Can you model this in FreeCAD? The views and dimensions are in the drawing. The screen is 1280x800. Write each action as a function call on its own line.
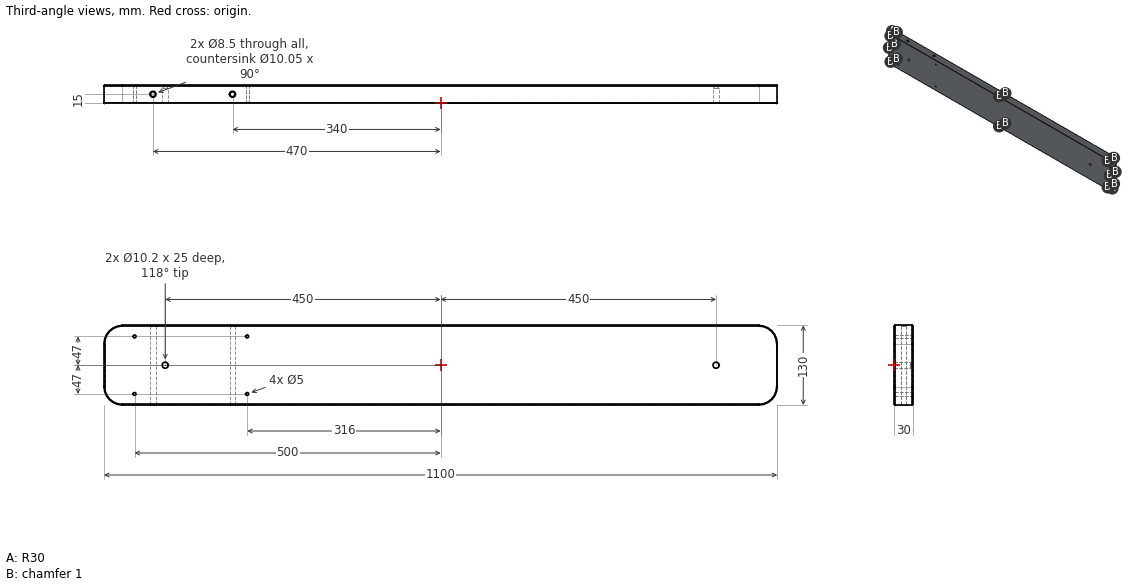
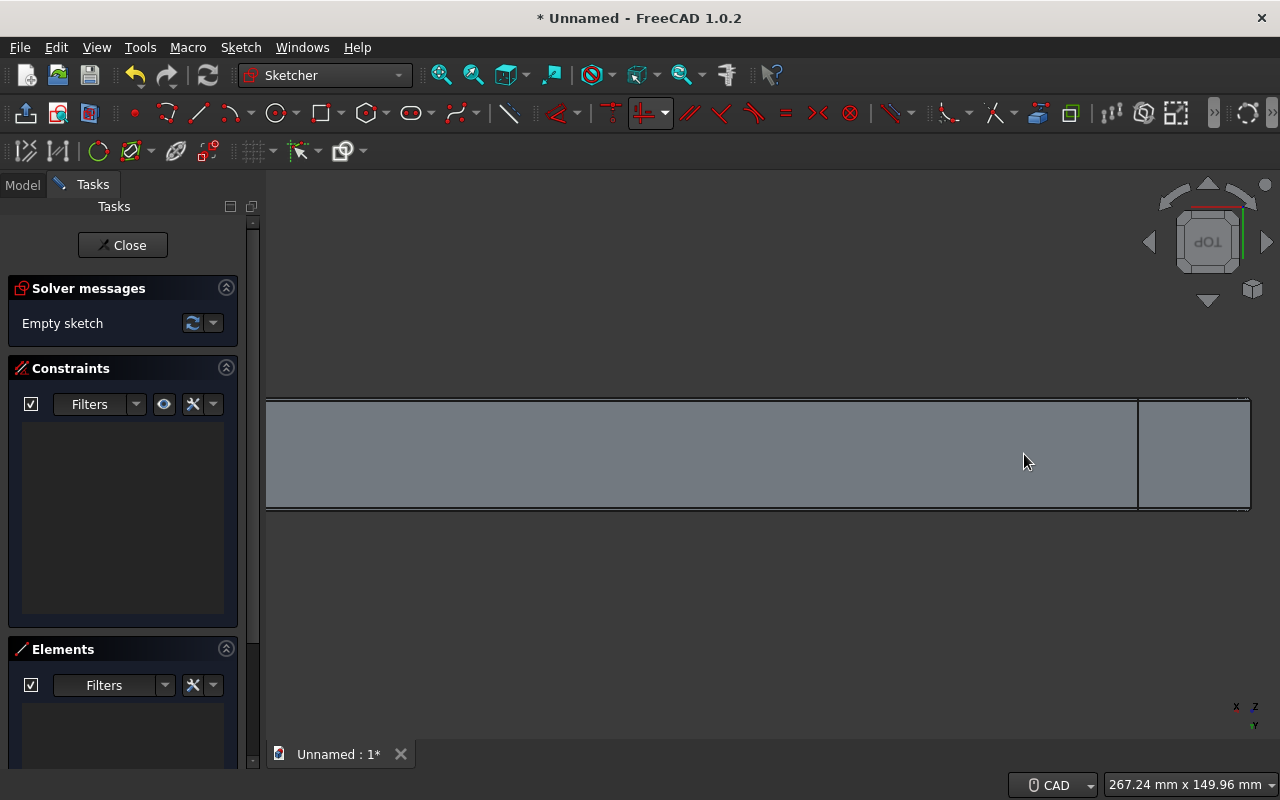
click(276, 114)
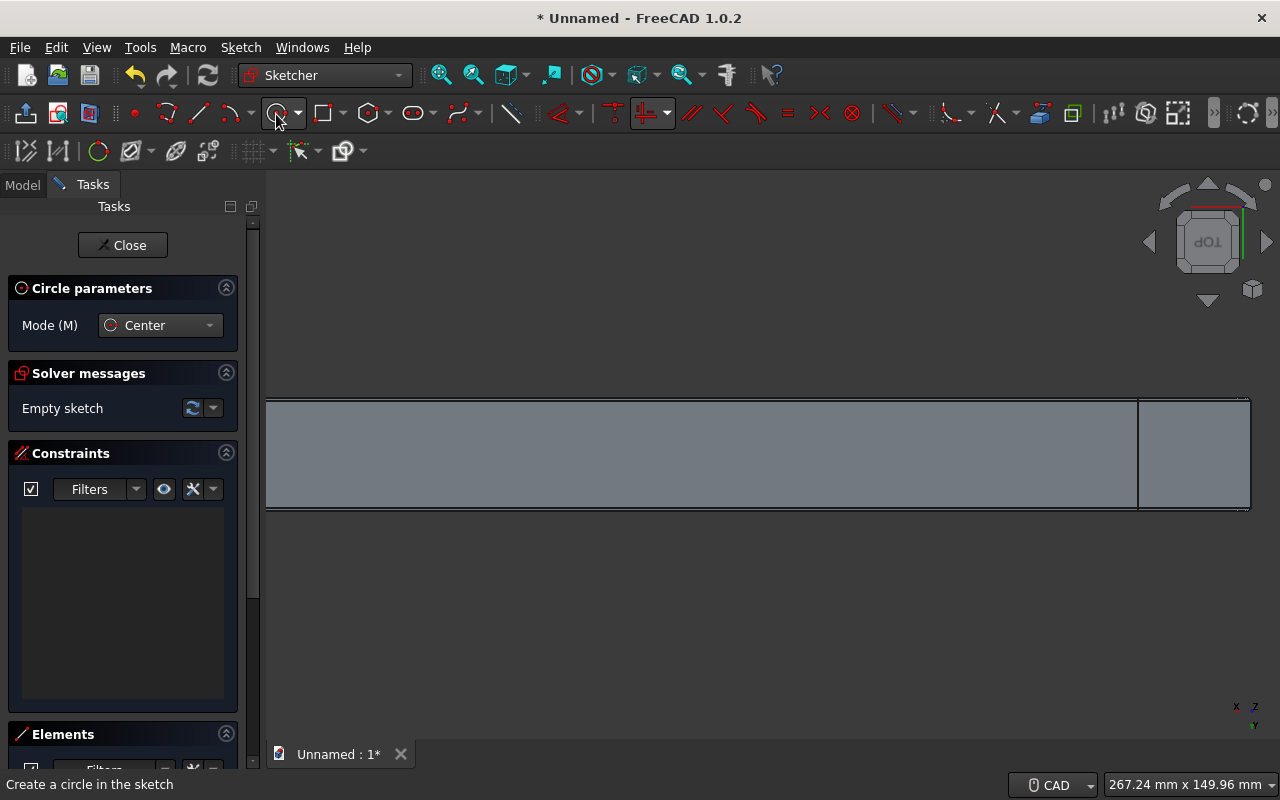
scroll(948, 455, up, 2)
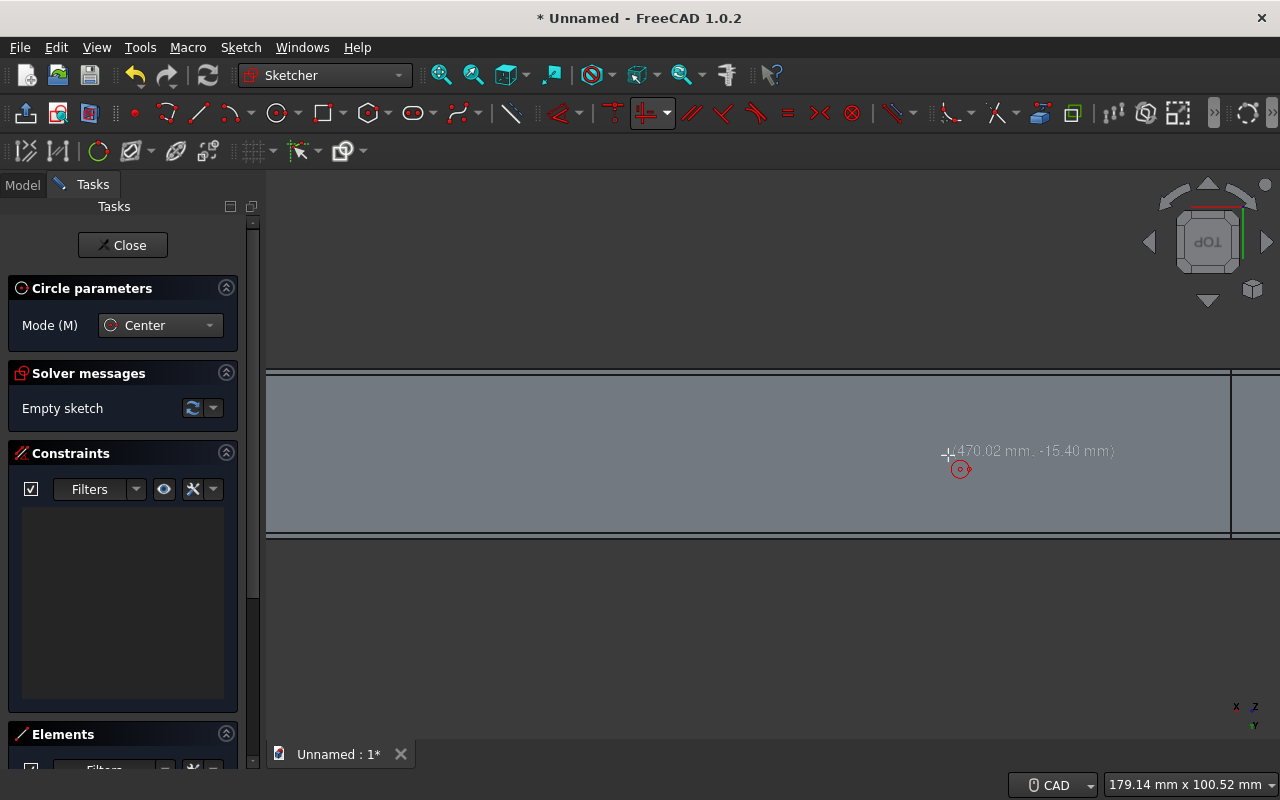
click(948, 454)
click(965, 437)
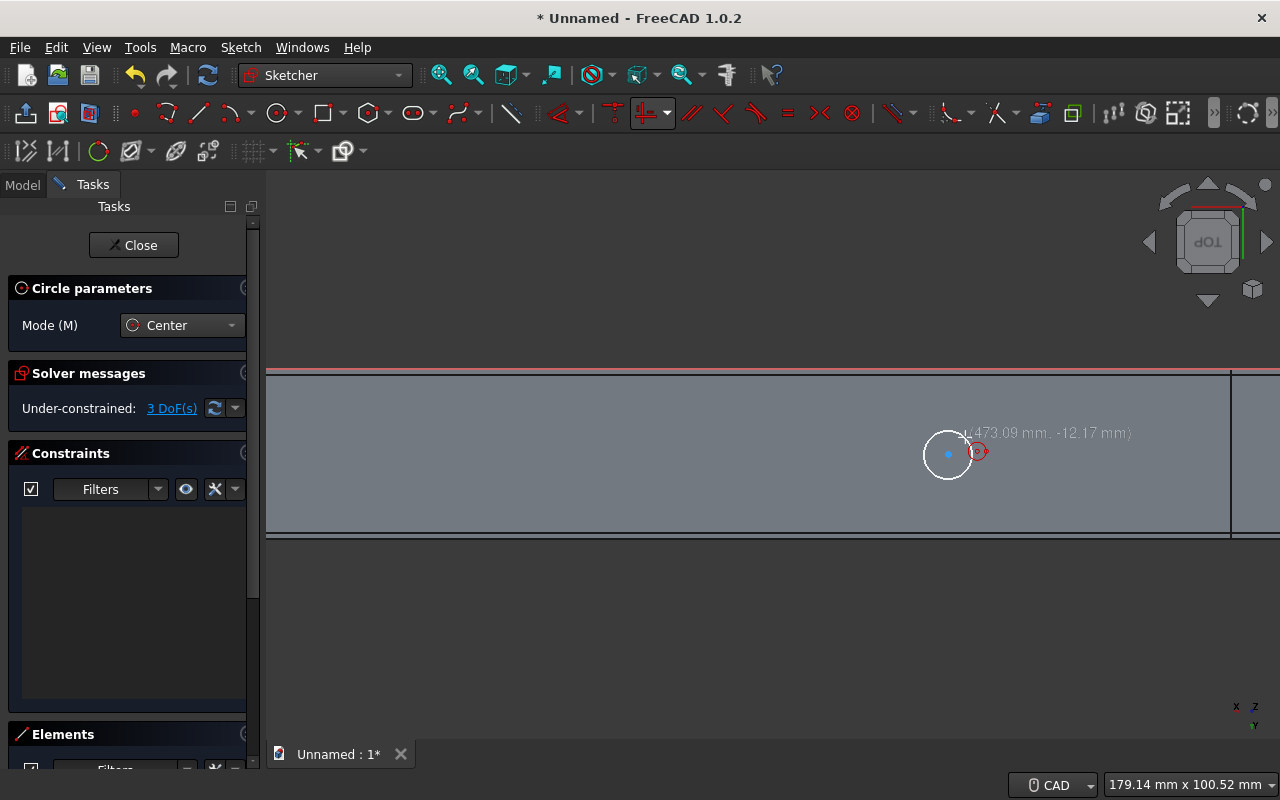
scroll(958, 456, down, 2)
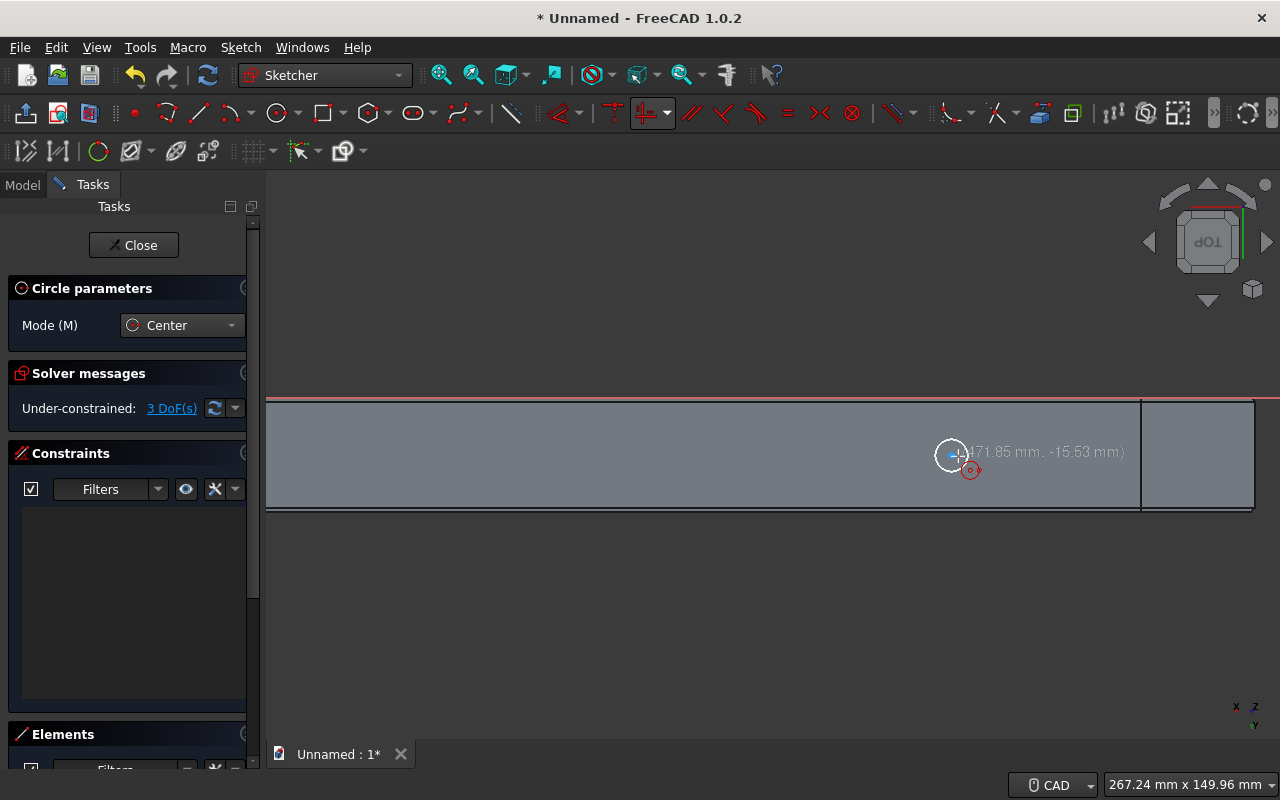
scroll(458, 455, up, 2)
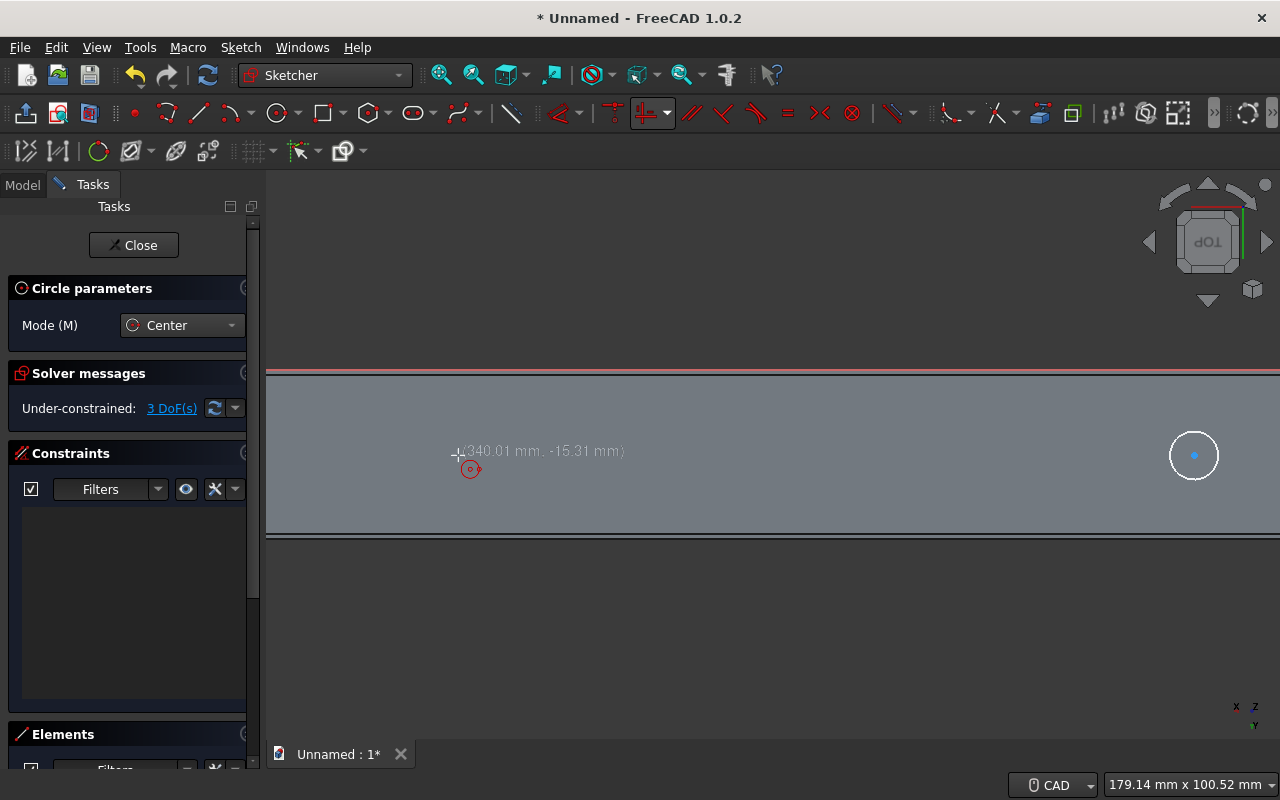
click(458, 454)
click(475, 437)
key(Escape)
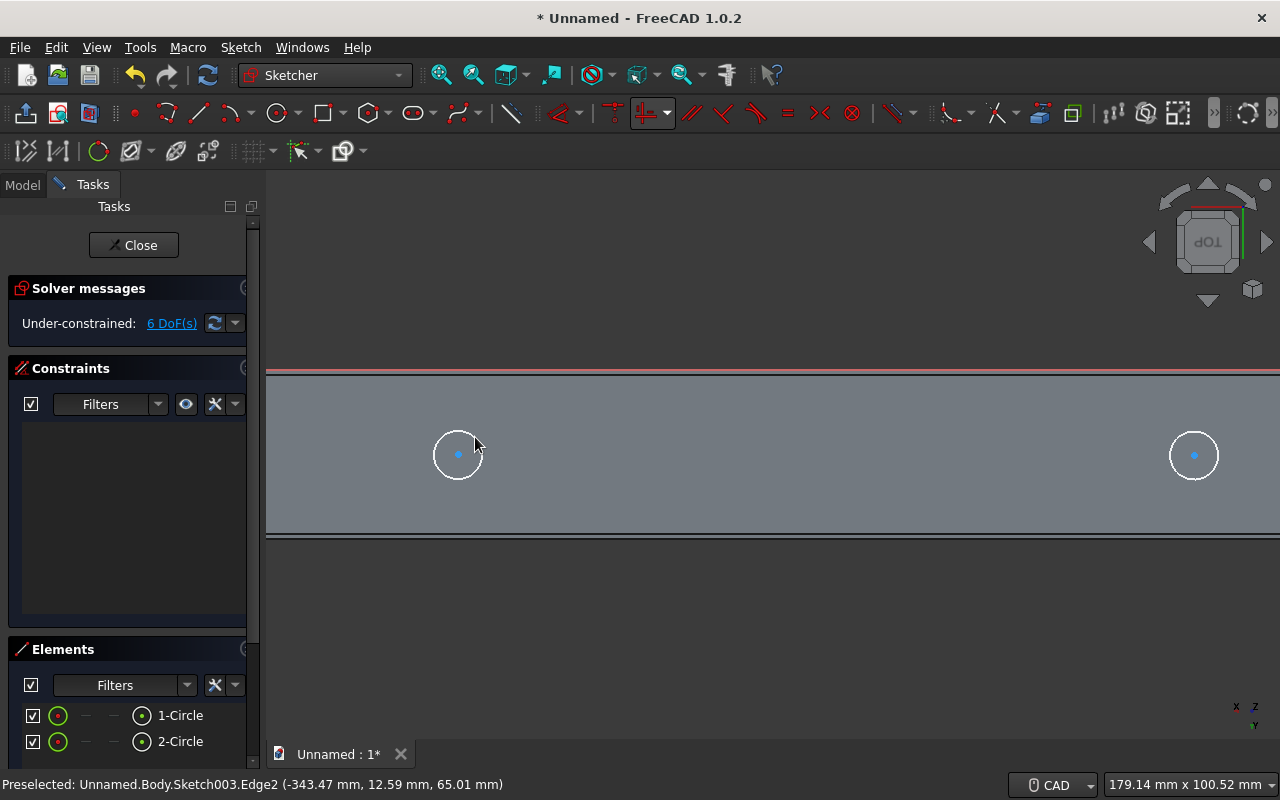
scroll(458, 455, down, 2)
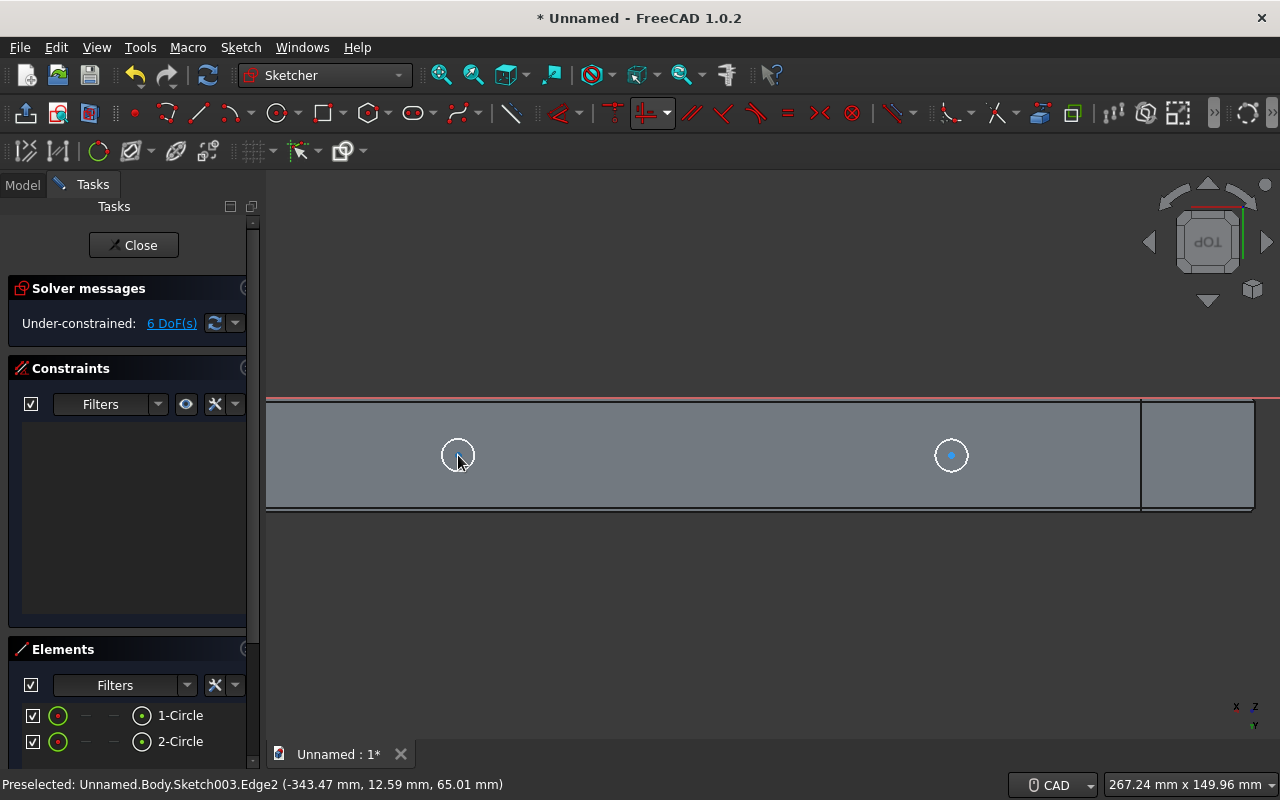
click(963, 444)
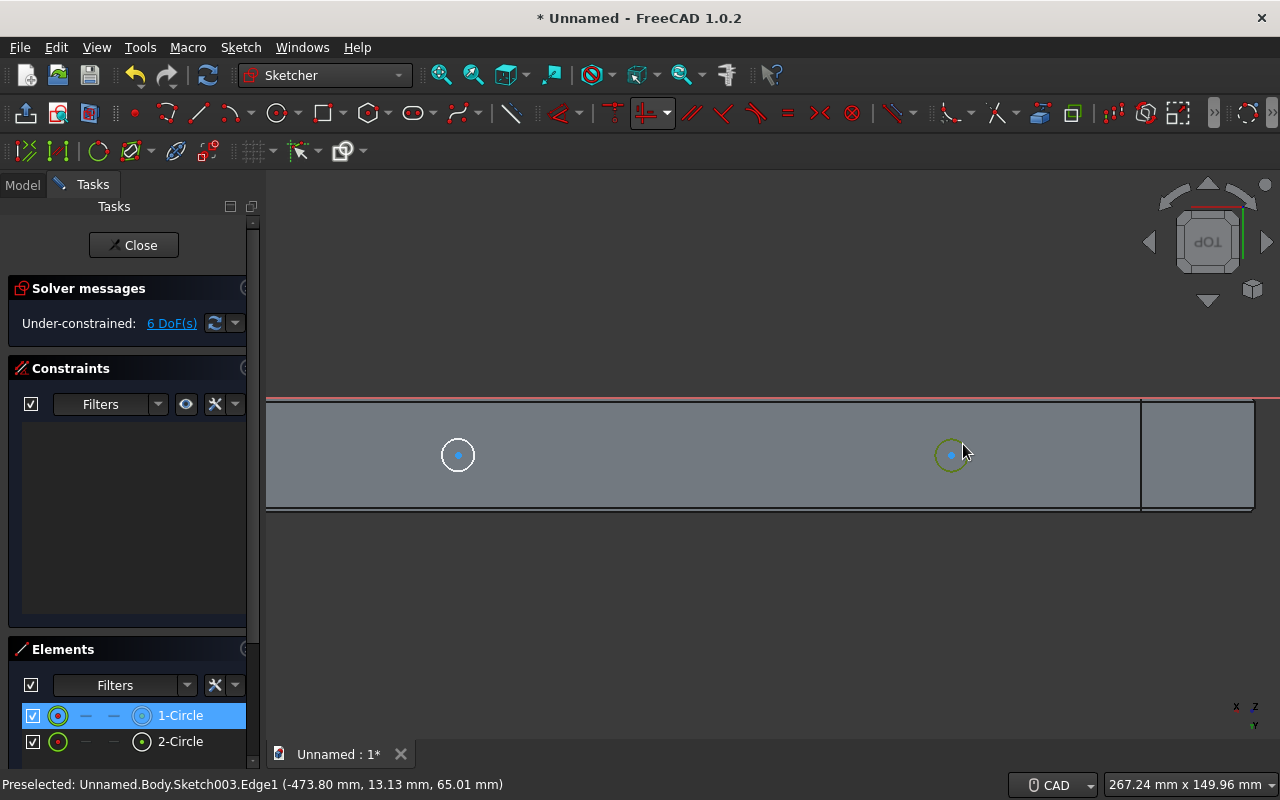
click(469, 444)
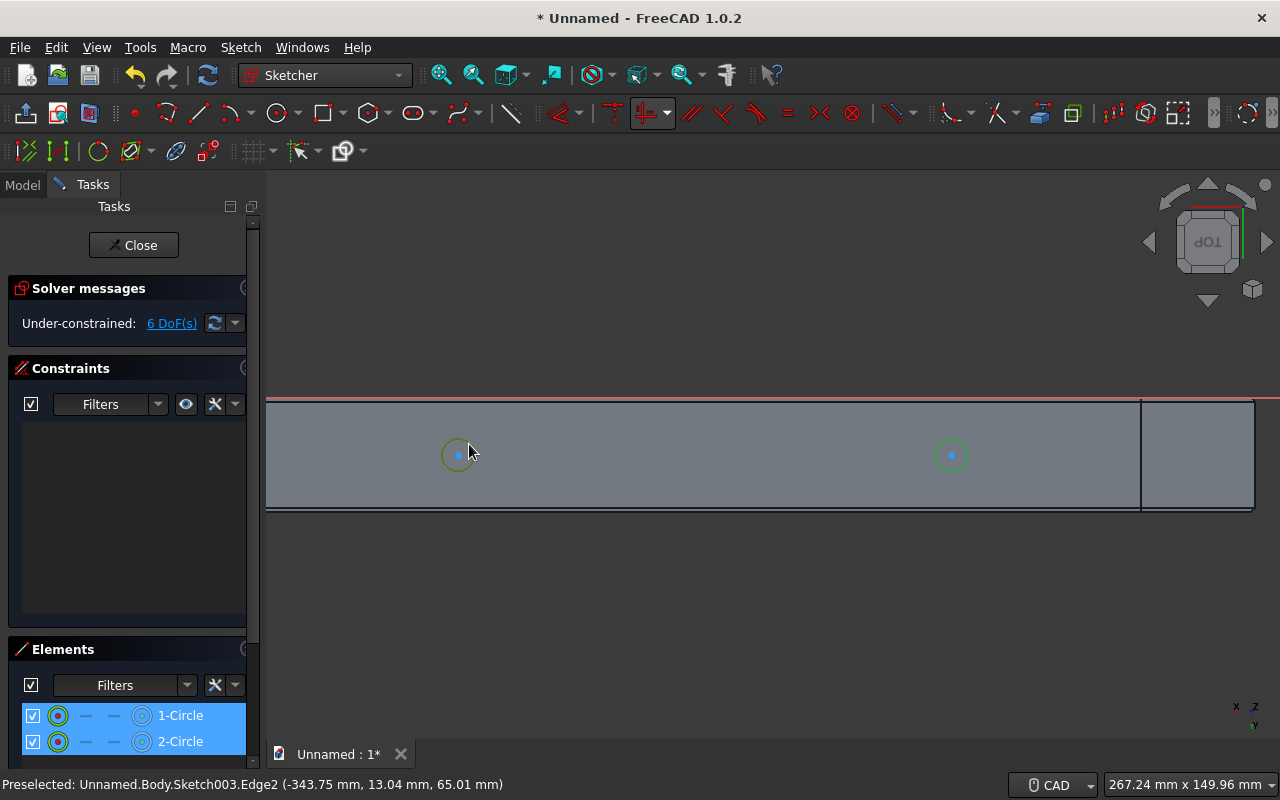
click(788, 114)